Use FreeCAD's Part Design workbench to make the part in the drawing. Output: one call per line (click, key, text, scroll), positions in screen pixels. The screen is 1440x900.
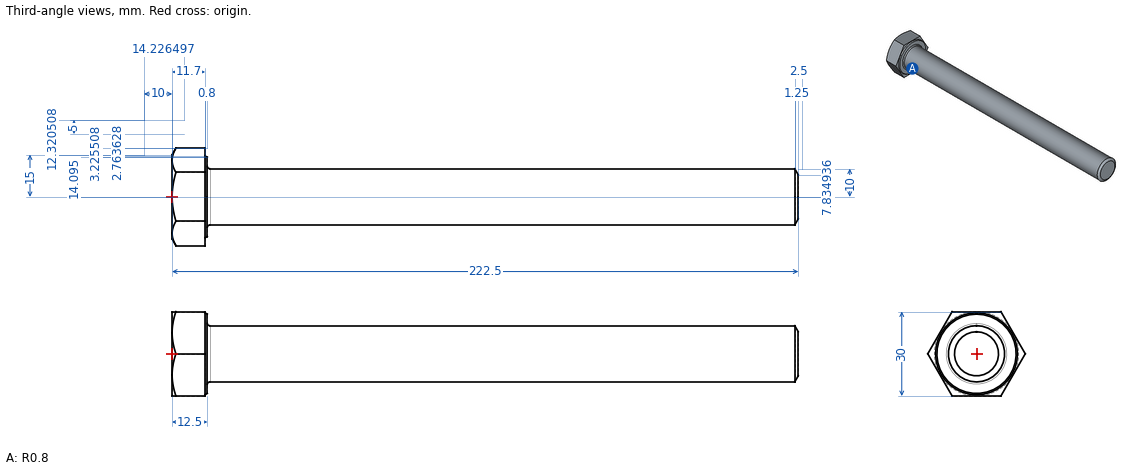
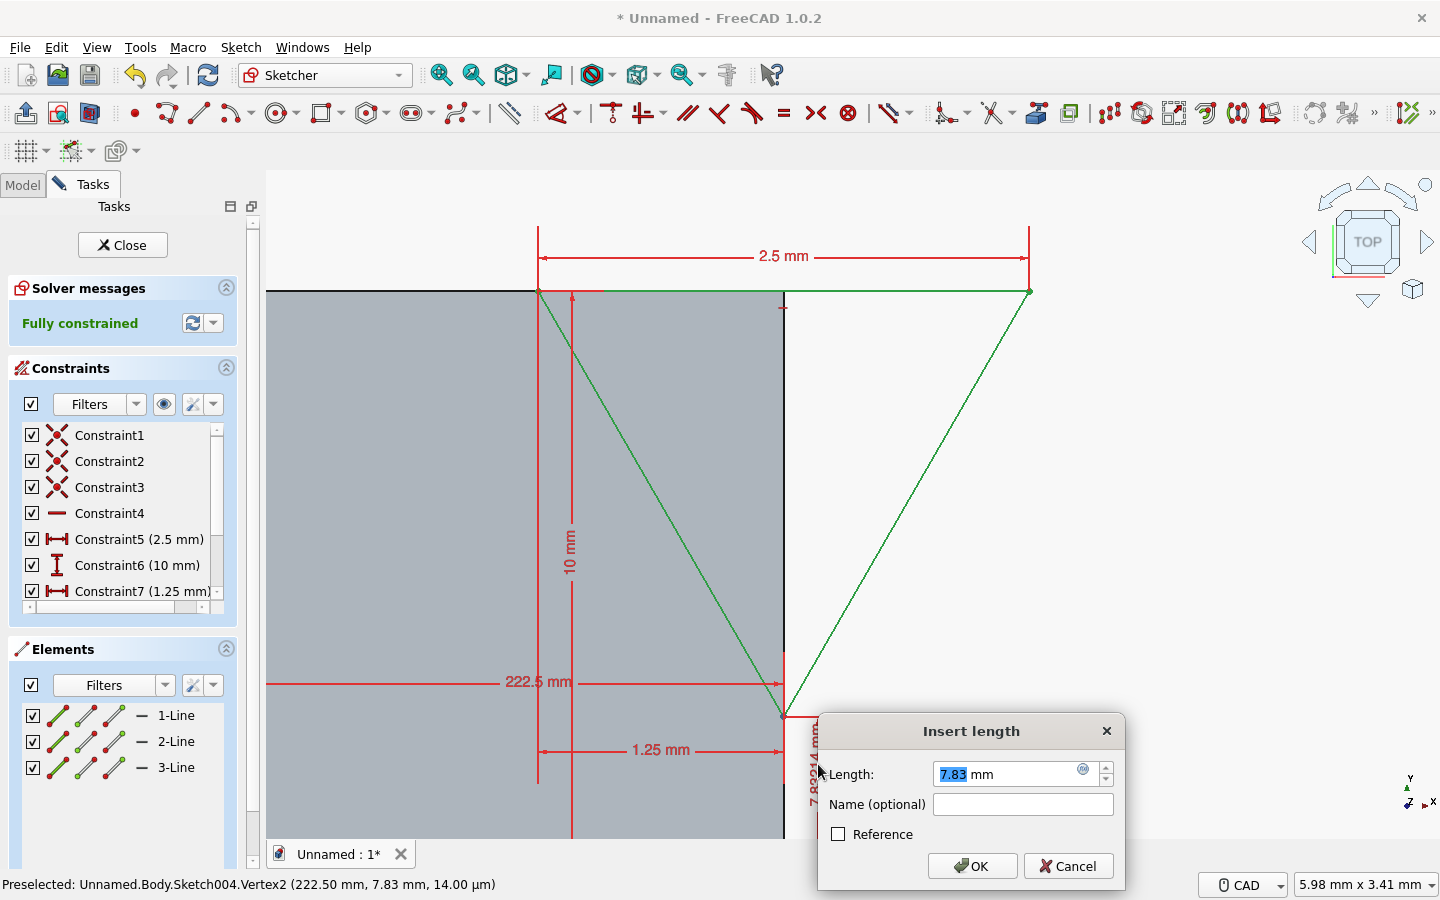
text(7.834936)
key(Return)
key(Escape)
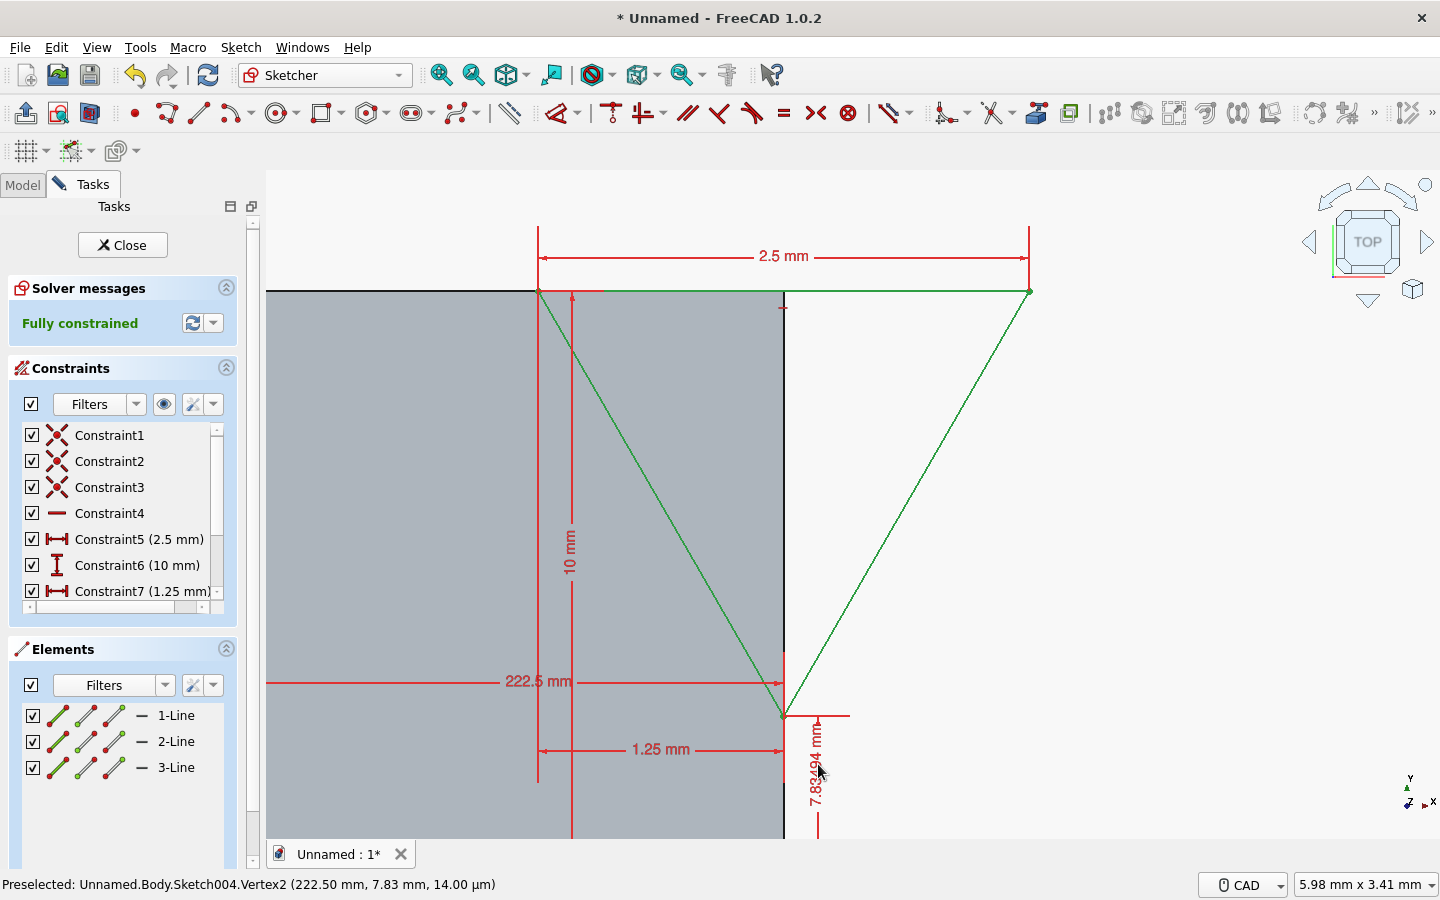
click(123, 245)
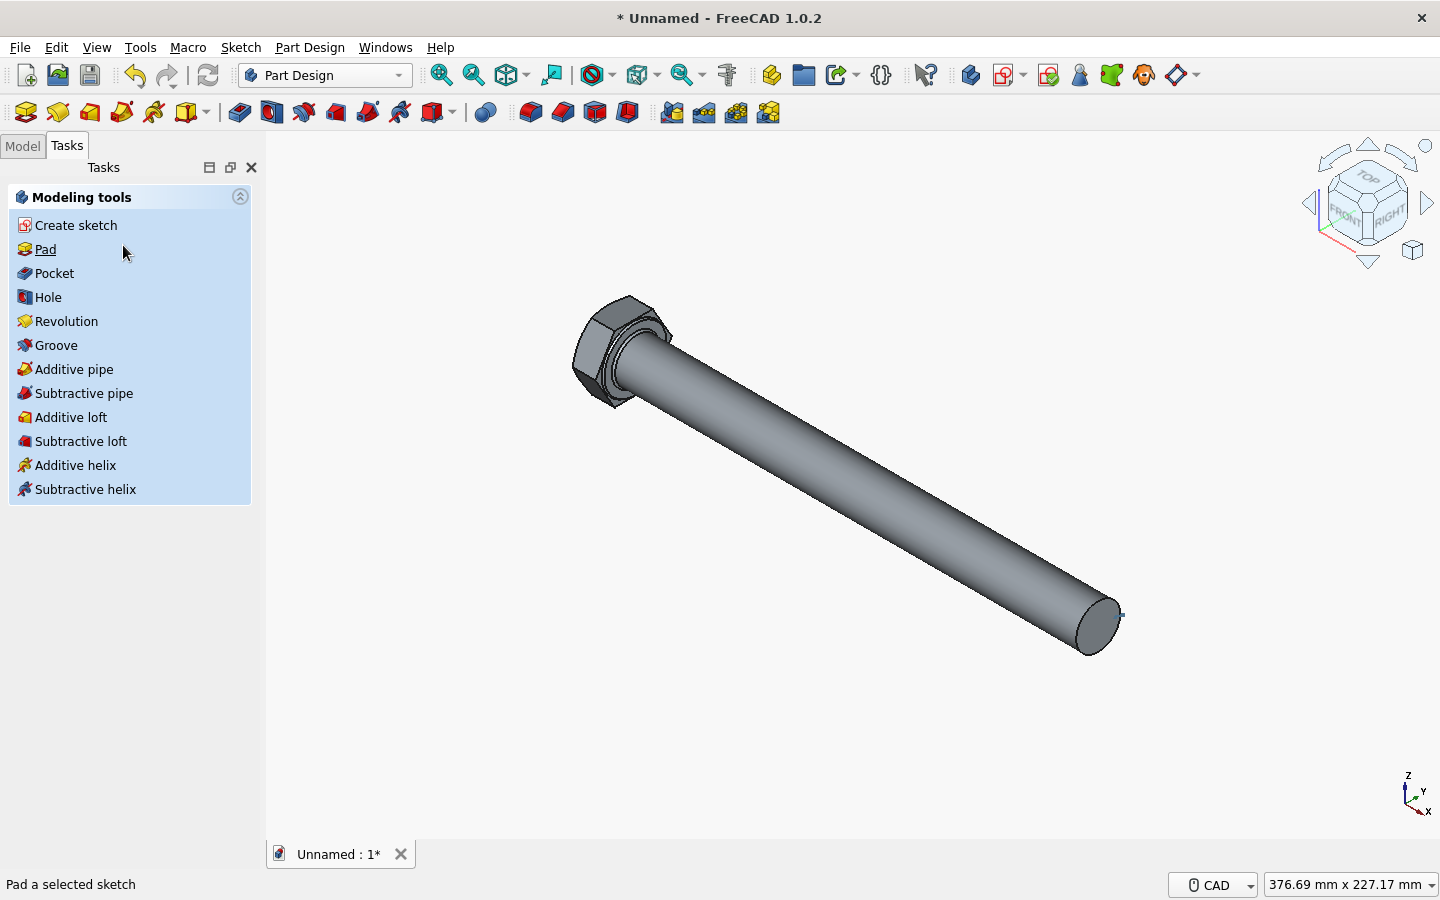
click(304, 112)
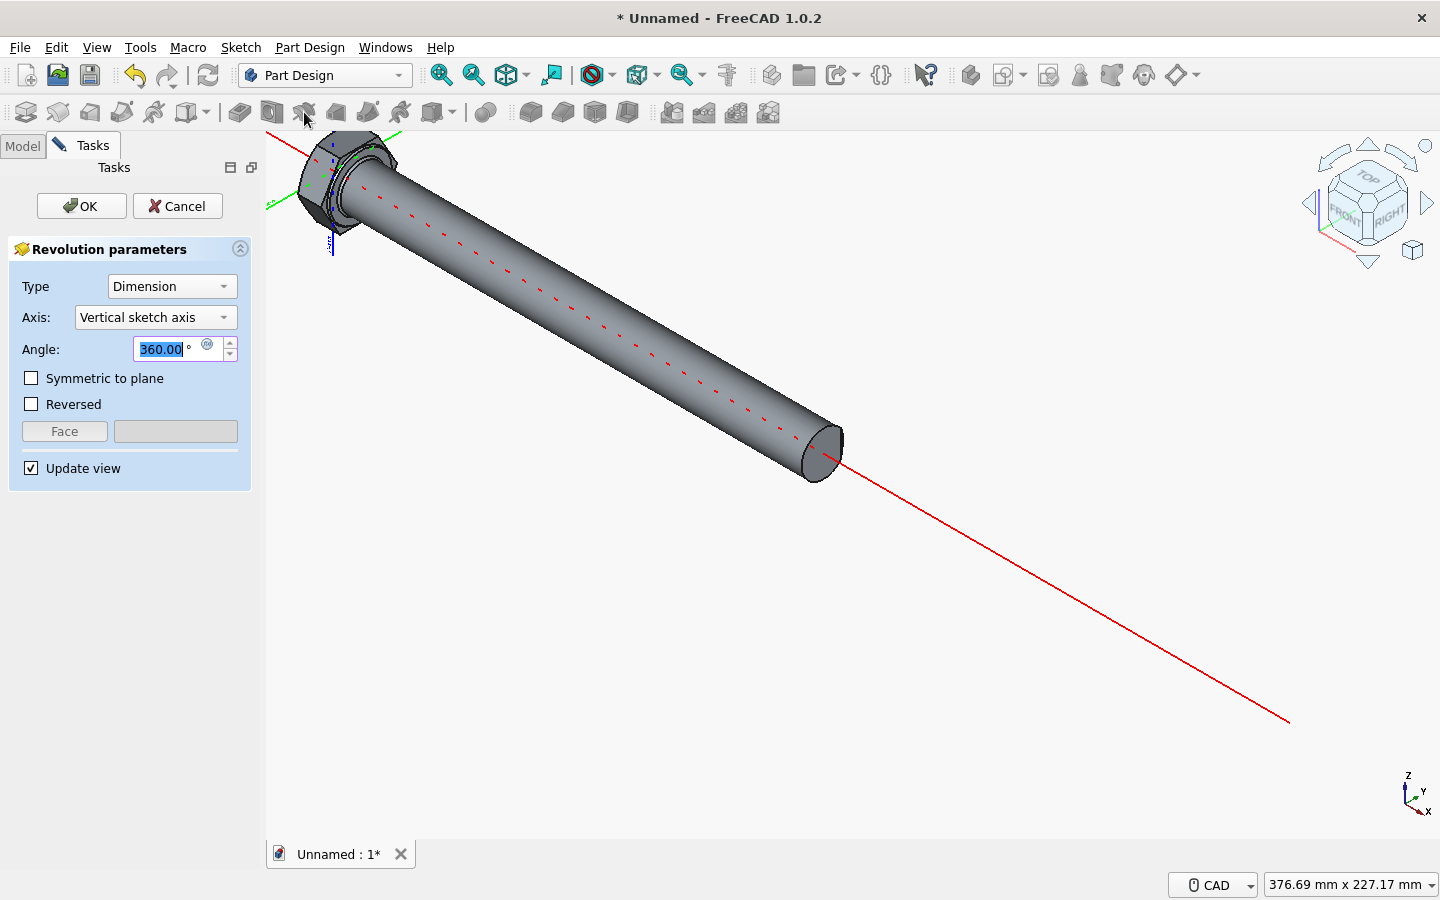
click(156, 318)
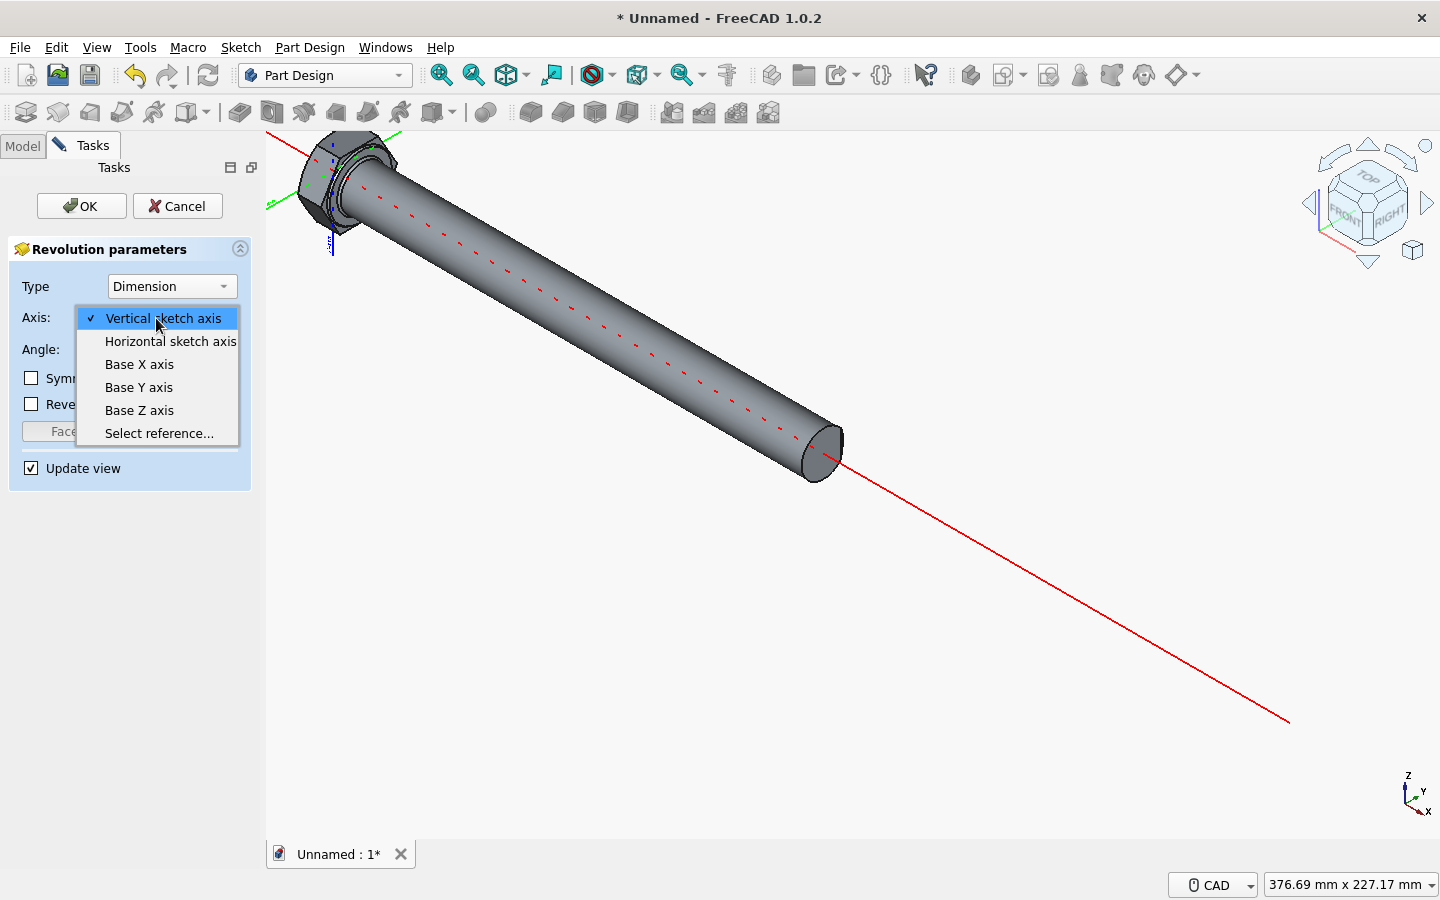
click(156, 342)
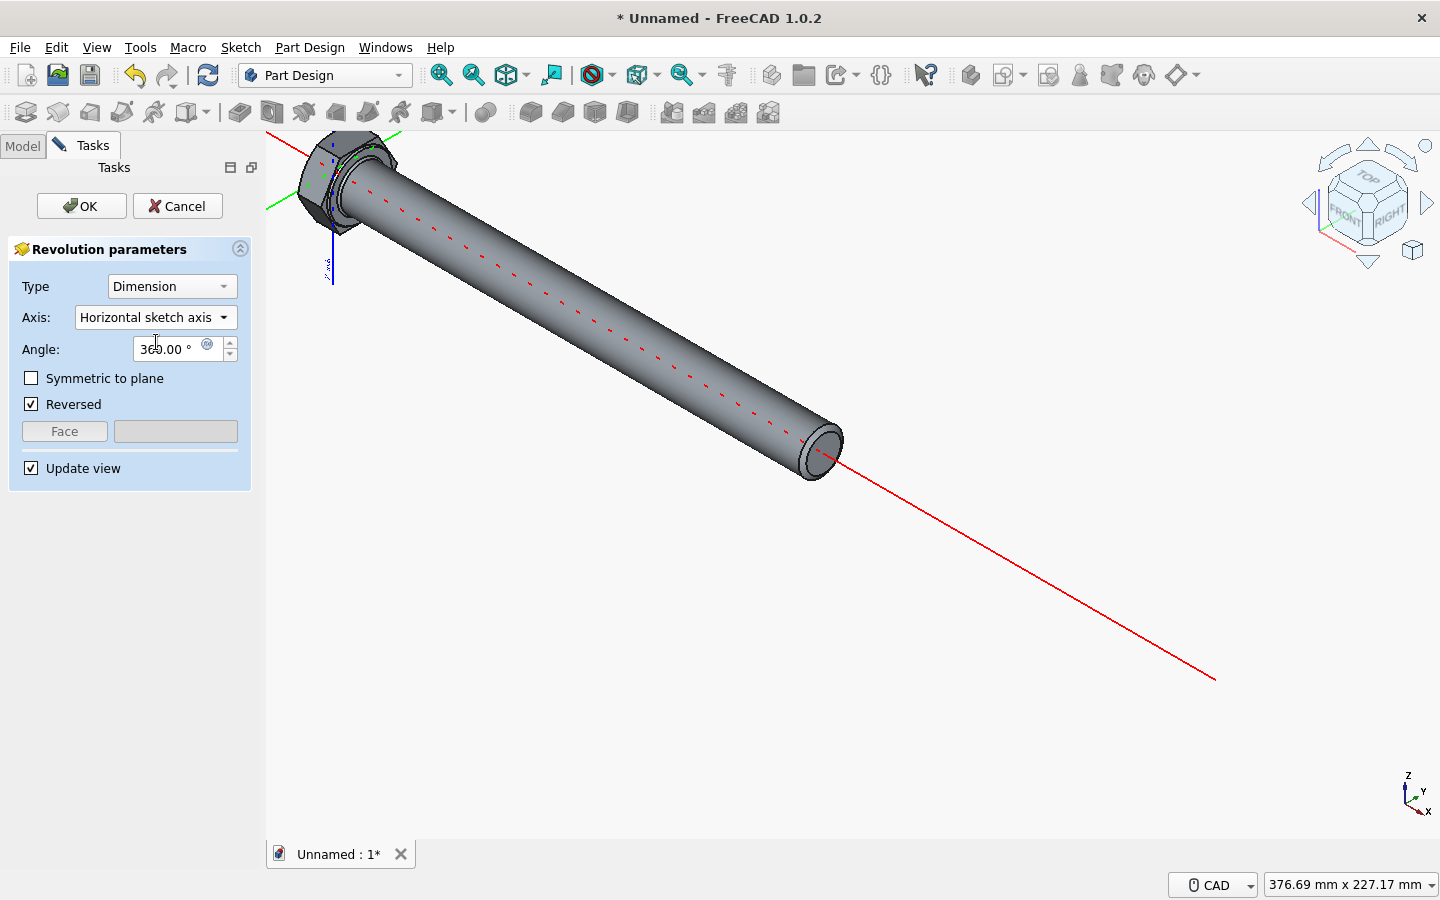
click(82, 206)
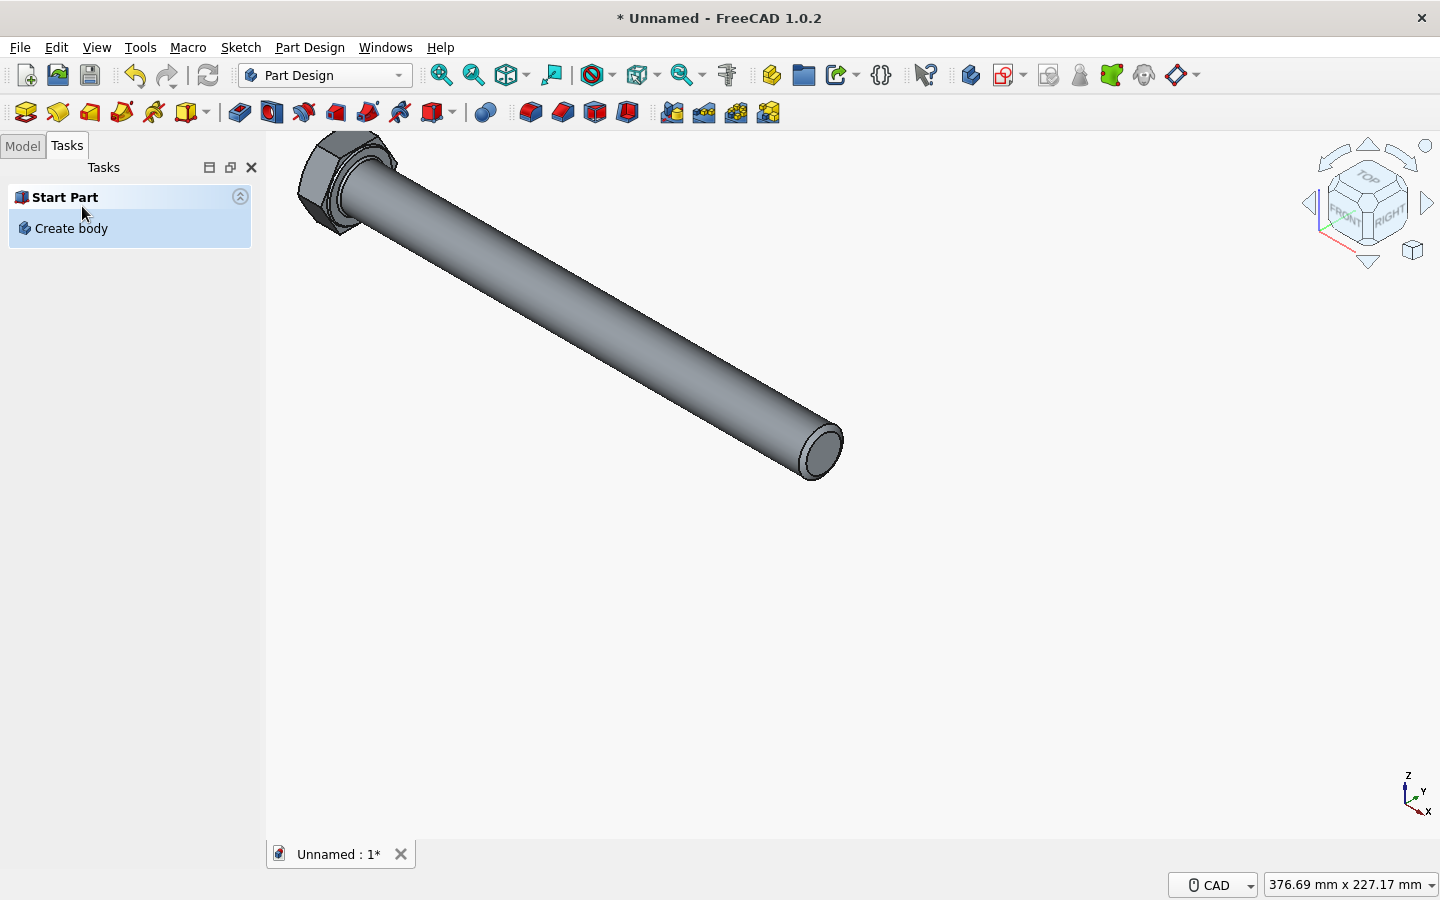
click(442, 76)